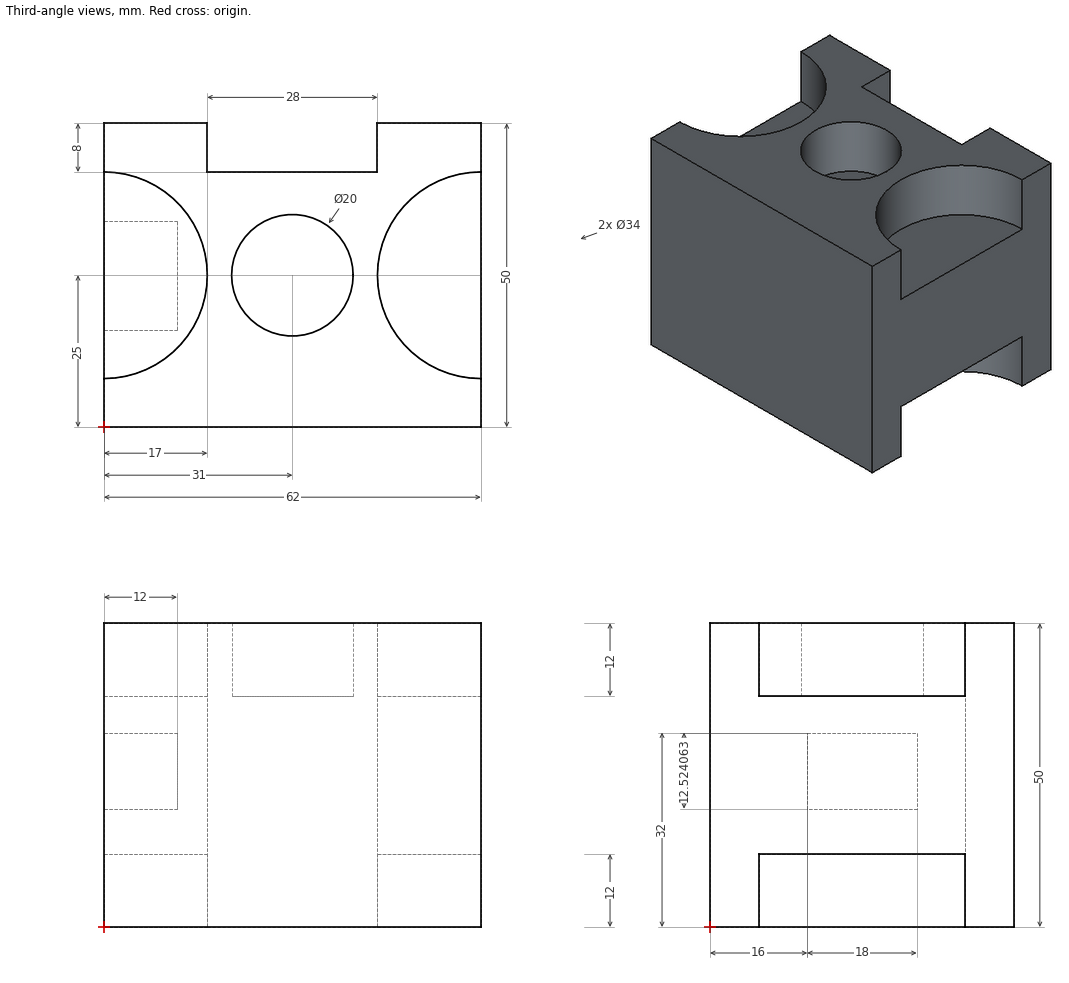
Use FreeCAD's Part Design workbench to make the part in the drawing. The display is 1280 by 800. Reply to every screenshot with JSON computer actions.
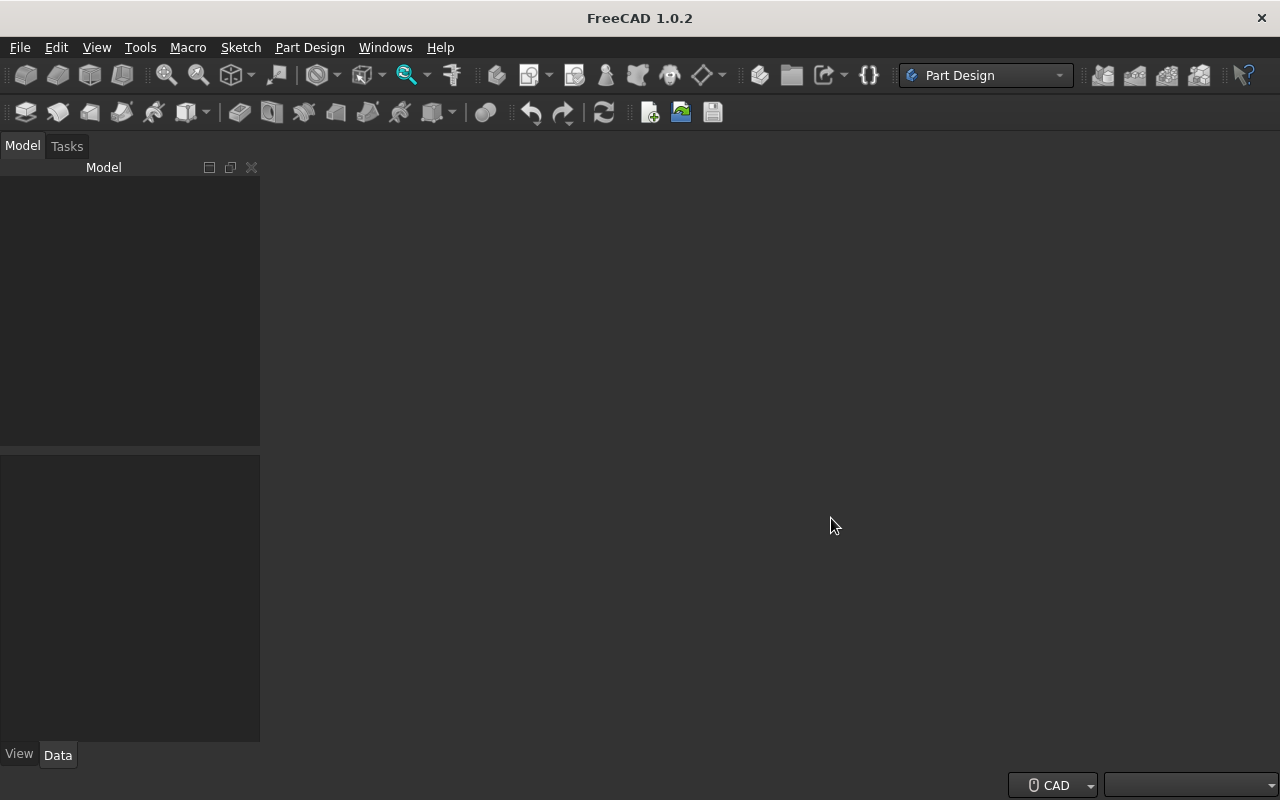
{"action": "left_click", "coordinate": [650, 112]}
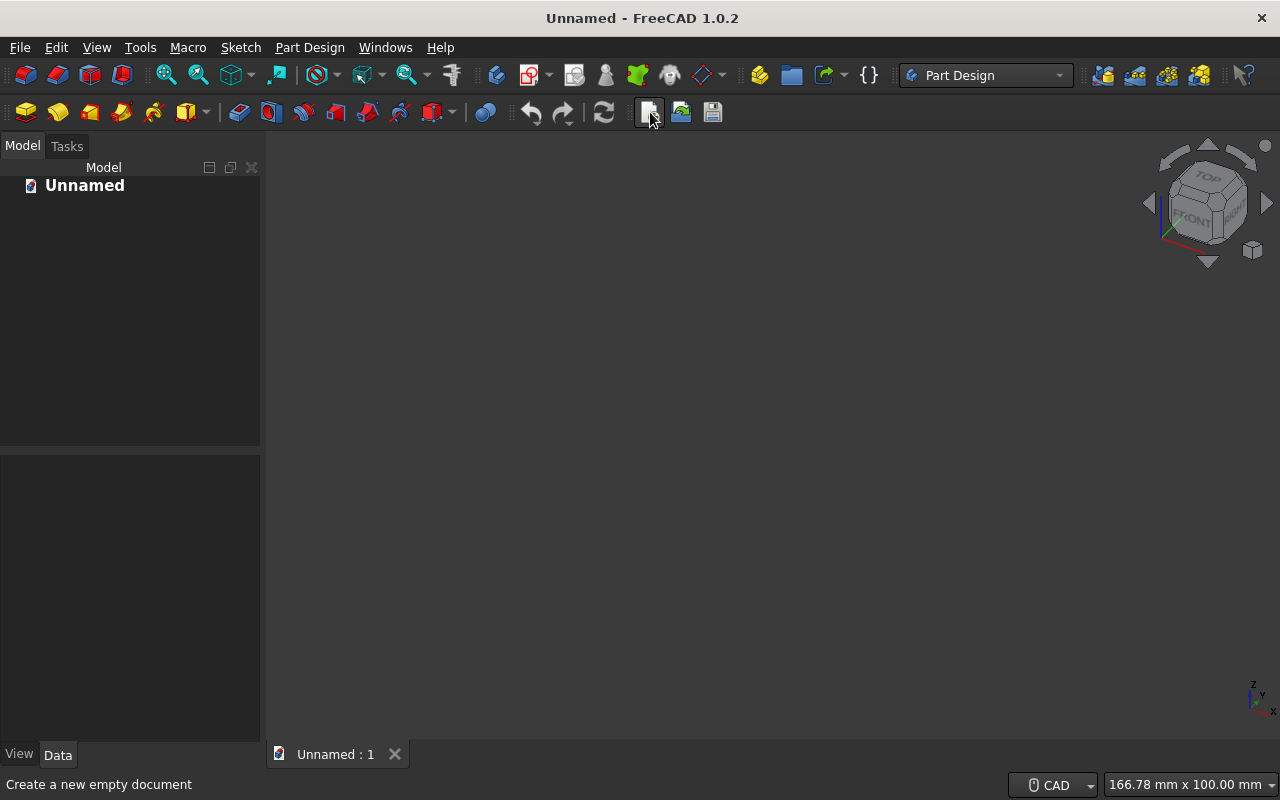
{"action": "left_click", "coordinate": [530, 76]}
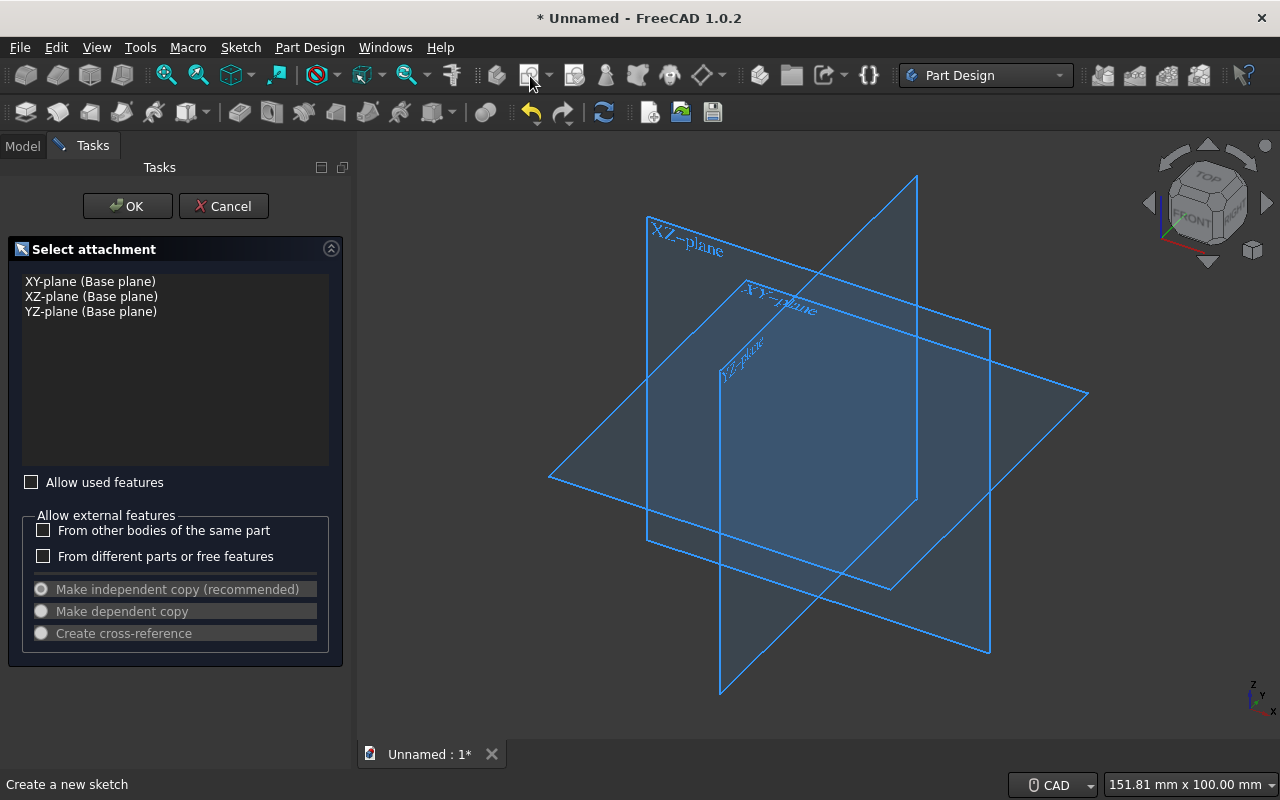
{"action": "left_click", "coordinate": [82, 282]}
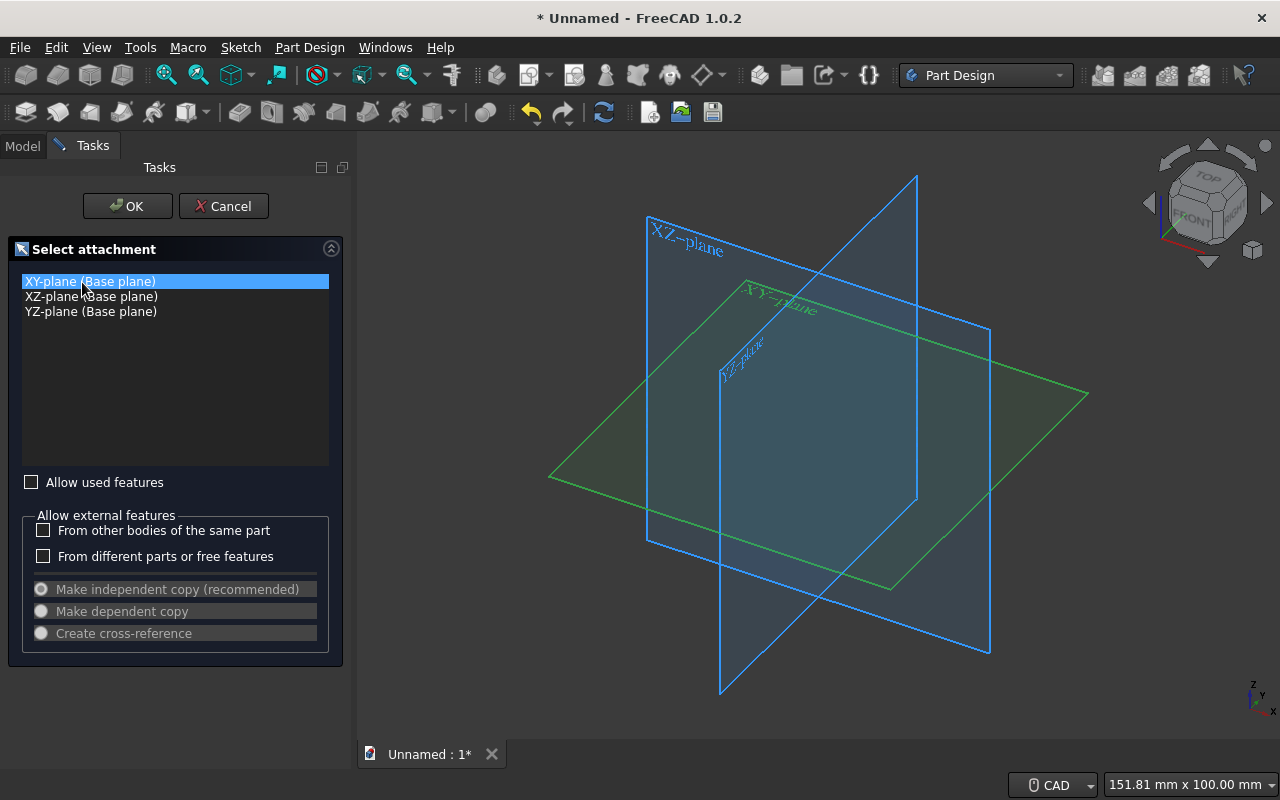
{"action": "left_click", "coordinate": [128, 206]}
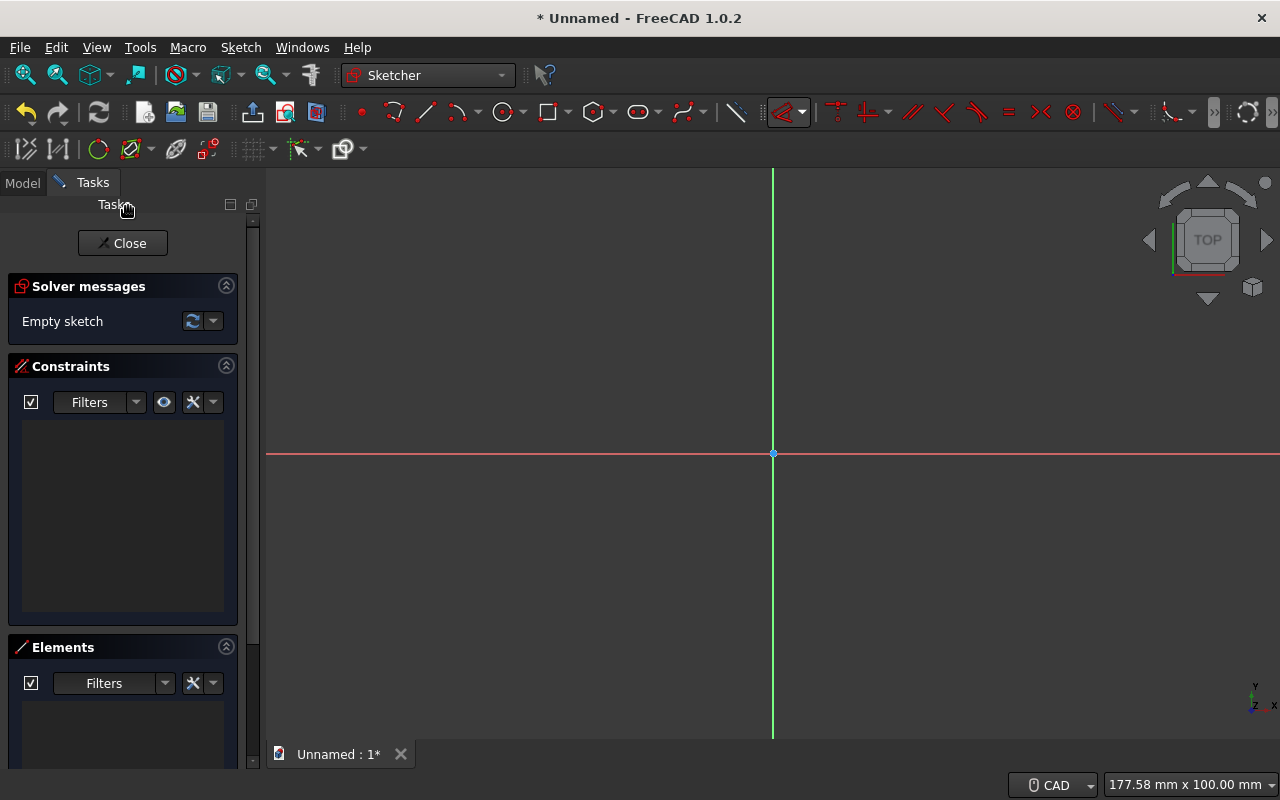
{"action": "scroll", "coordinate": [294, 711], "scroll_direction": "down", "scroll_amount": 1}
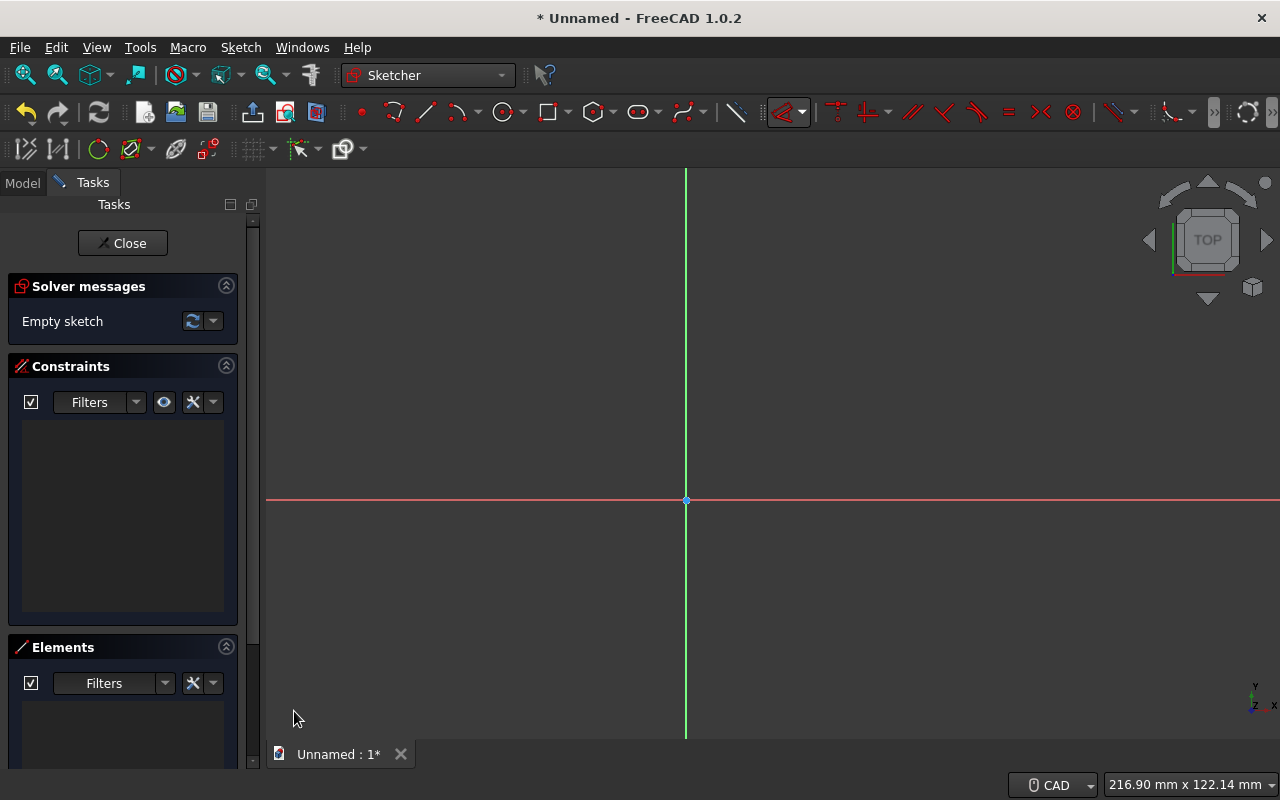
{"action": "scroll", "coordinate": [1089, 241], "scroll_direction": "up", "scroll_amount": 2}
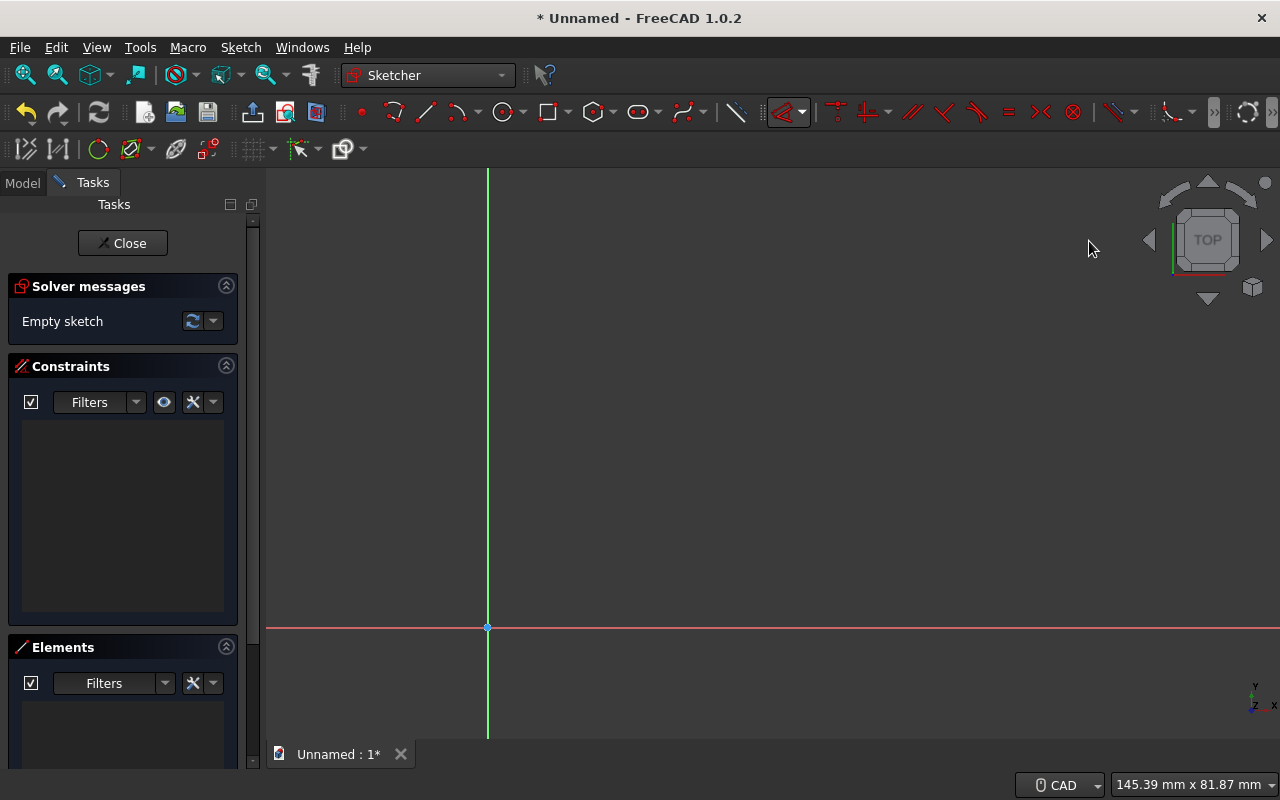
{"action": "left_click", "coordinate": [548, 112]}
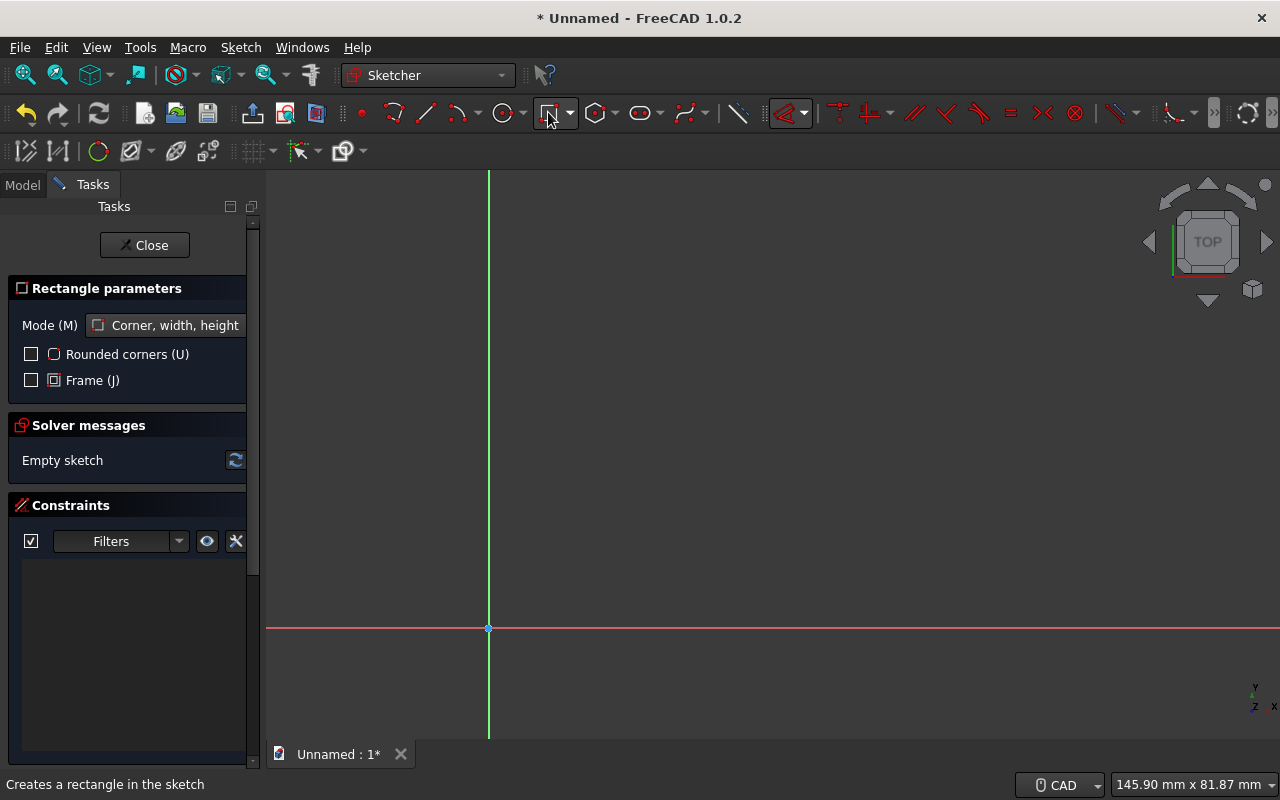
{"action": "left_click", "coordinate": [489, 628]}
{"action": "left_click", "coordinate": [920, 281]}
{"action": "key", "text": "Escape"}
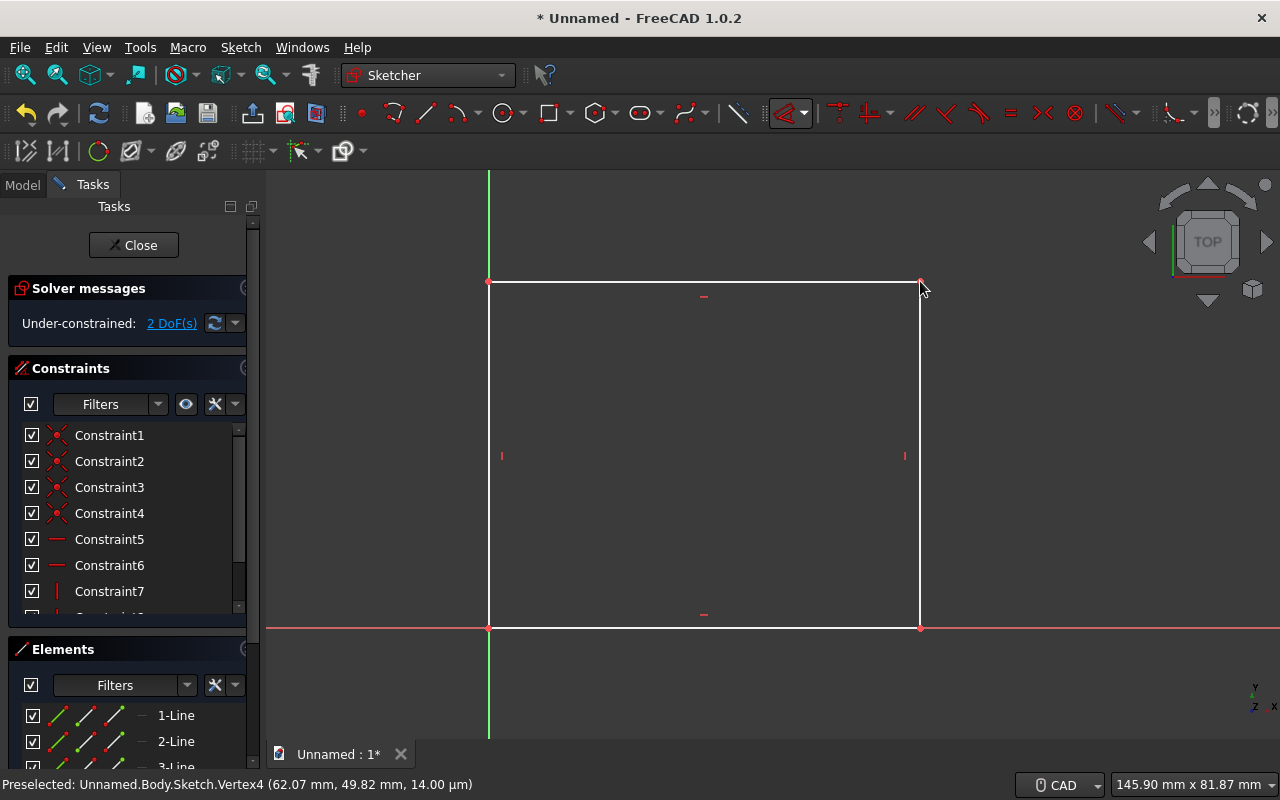
{"action": "left_click", "coordinate": [784, 114]}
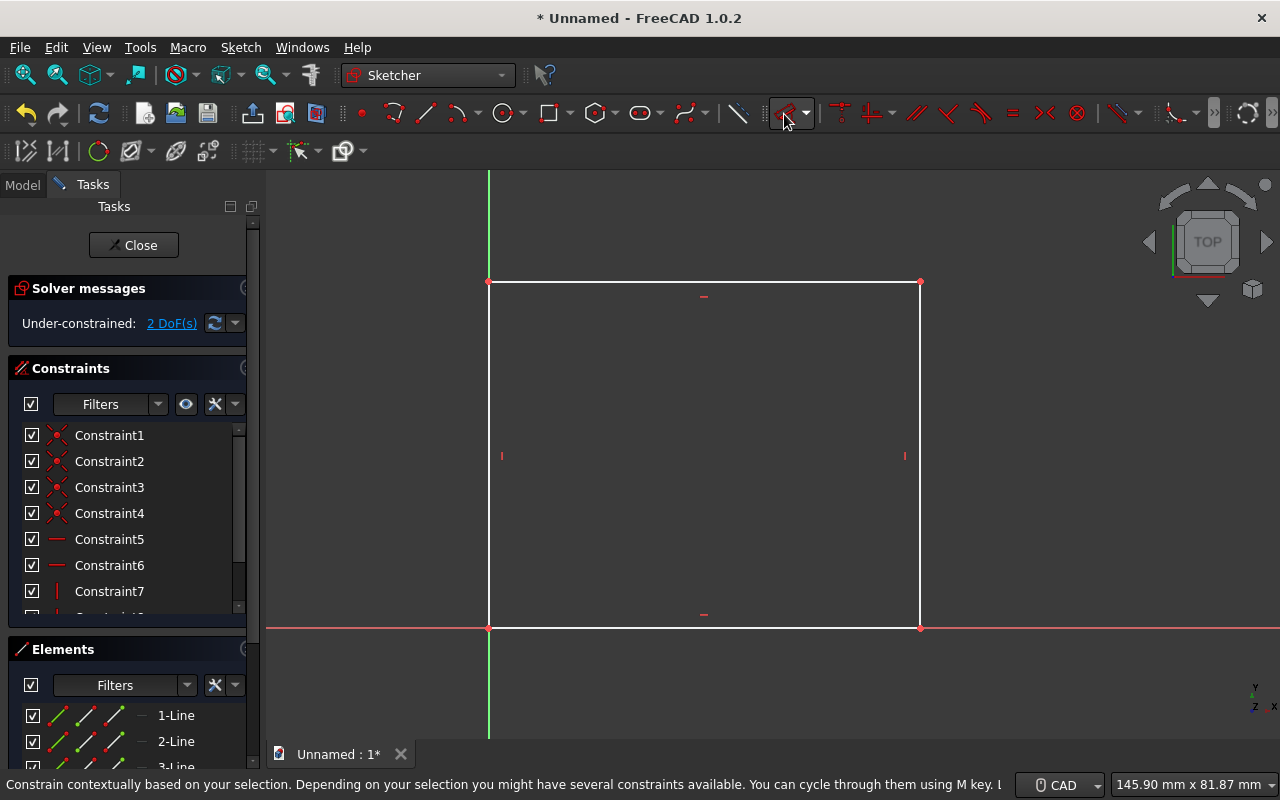
{"action": "left_click", "coordinate": [618, 628]}
{"action": "left_click", "coordinate": [704, 662]}